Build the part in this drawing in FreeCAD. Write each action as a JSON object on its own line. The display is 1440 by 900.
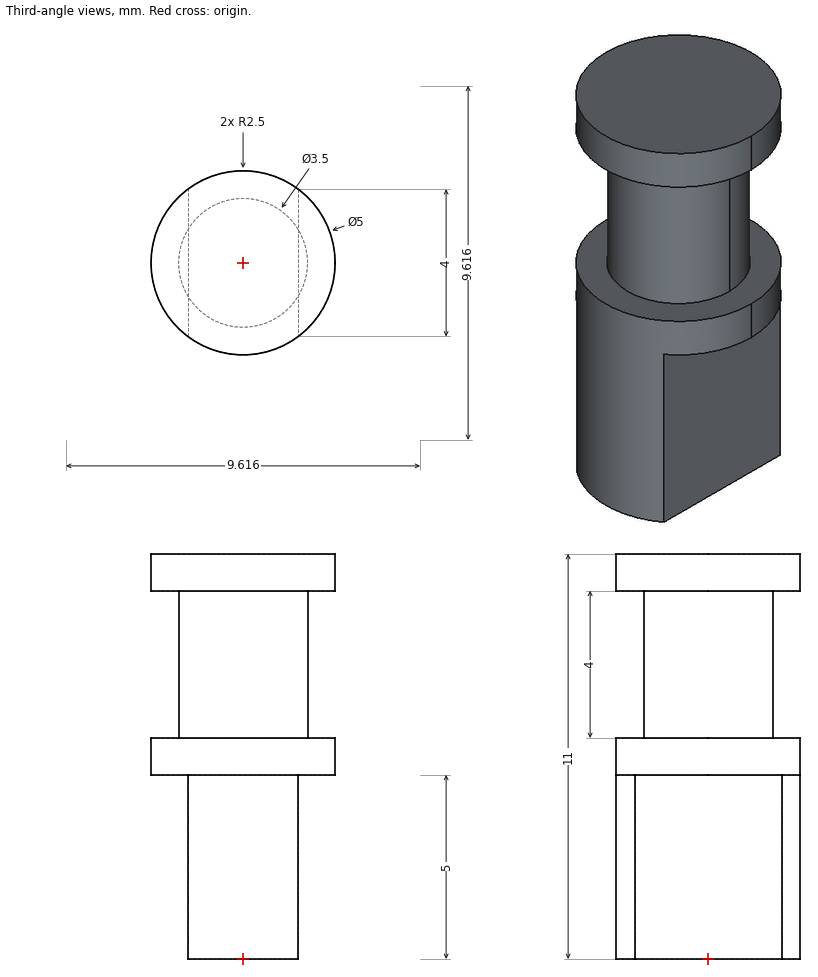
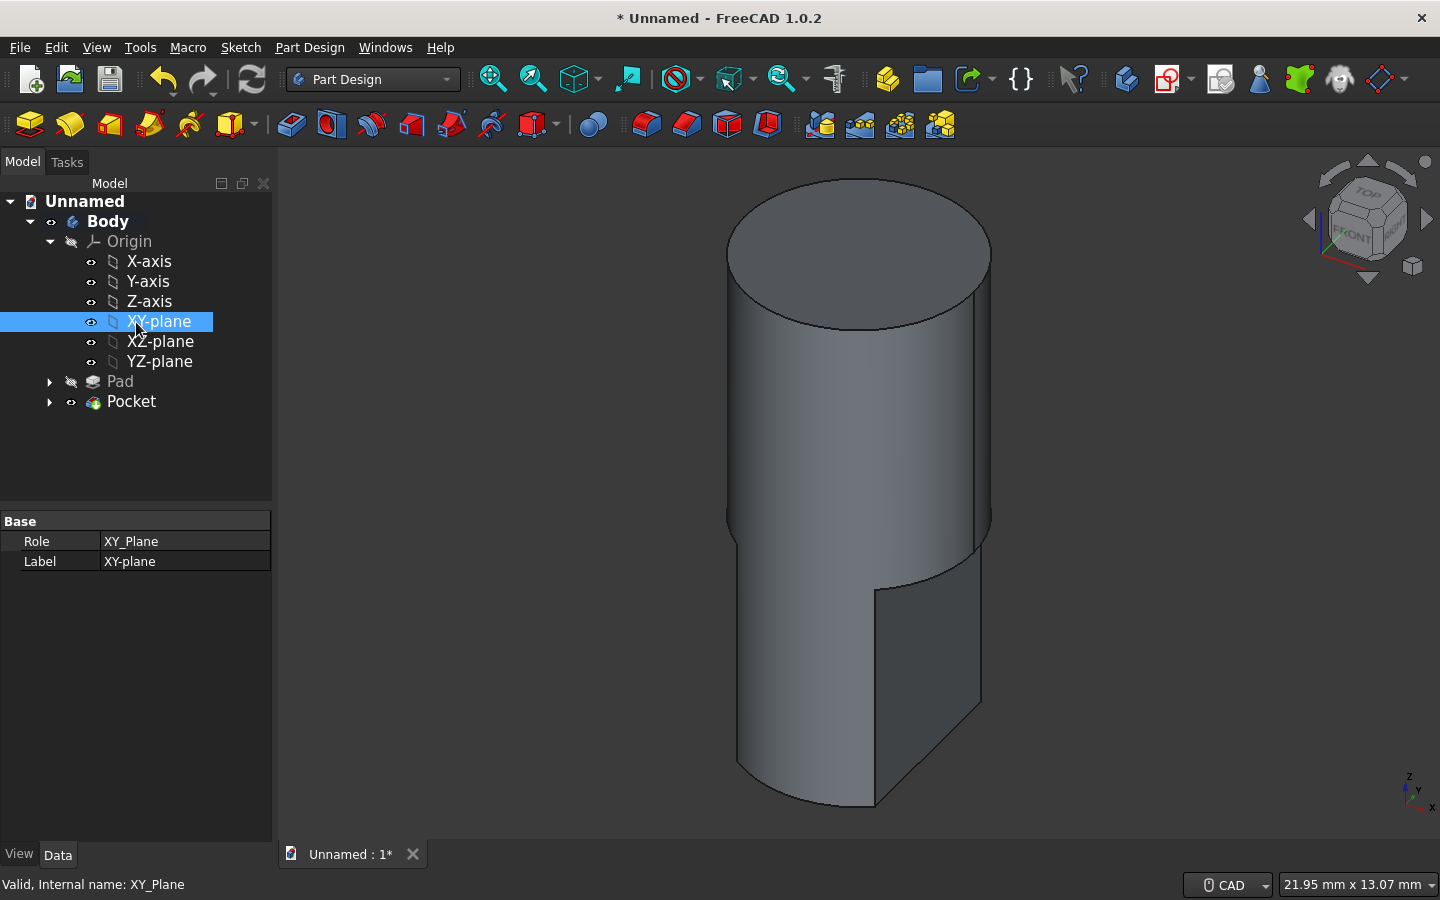
{"action": "left_click", "coordinate": [1380, 80]}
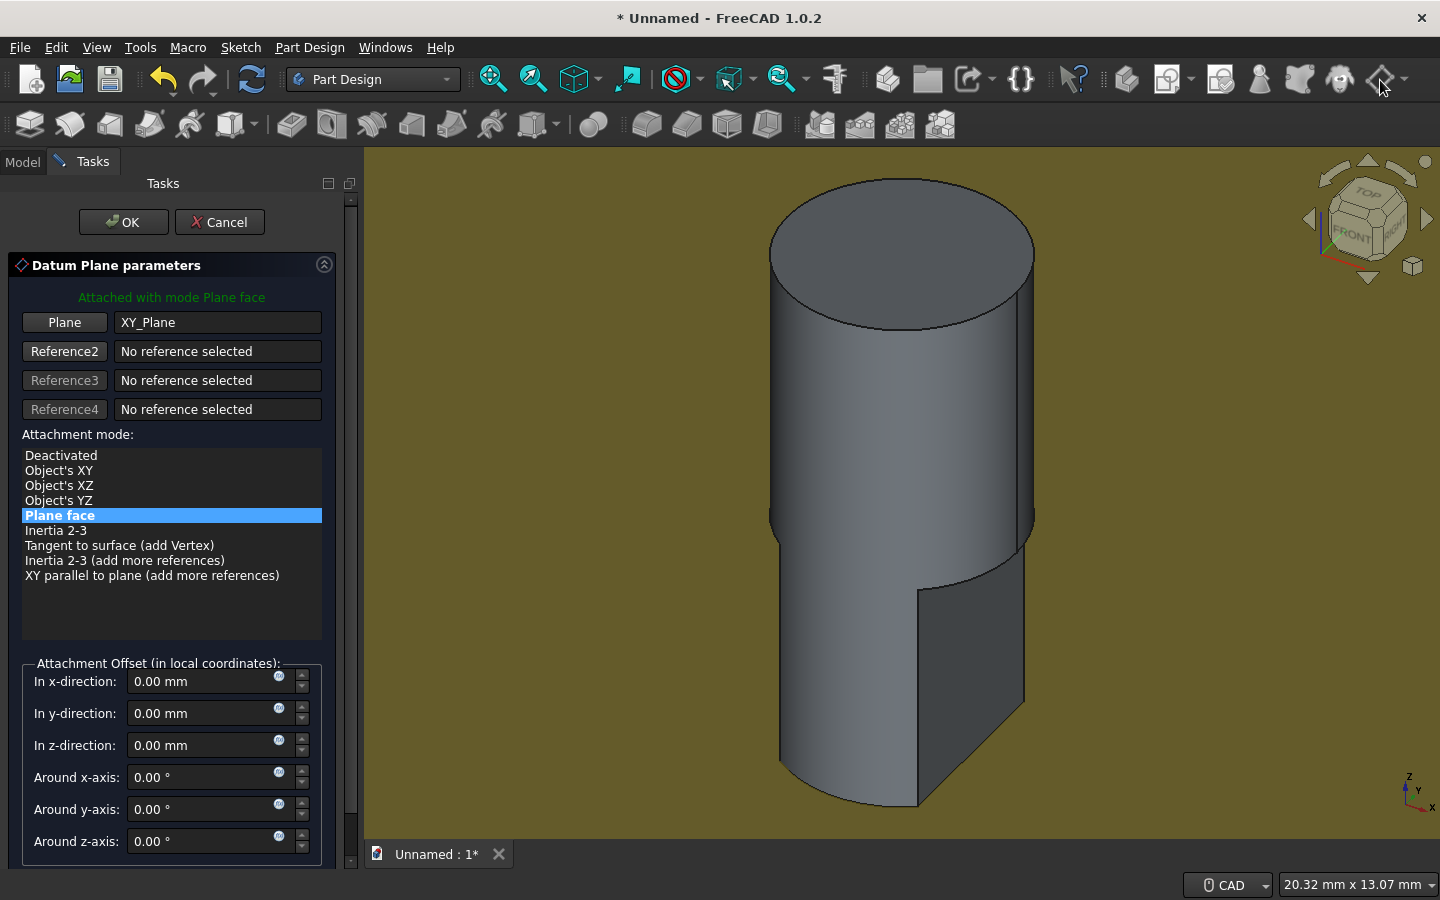
{"action": "triple_click", "coordinate": [210, 745]}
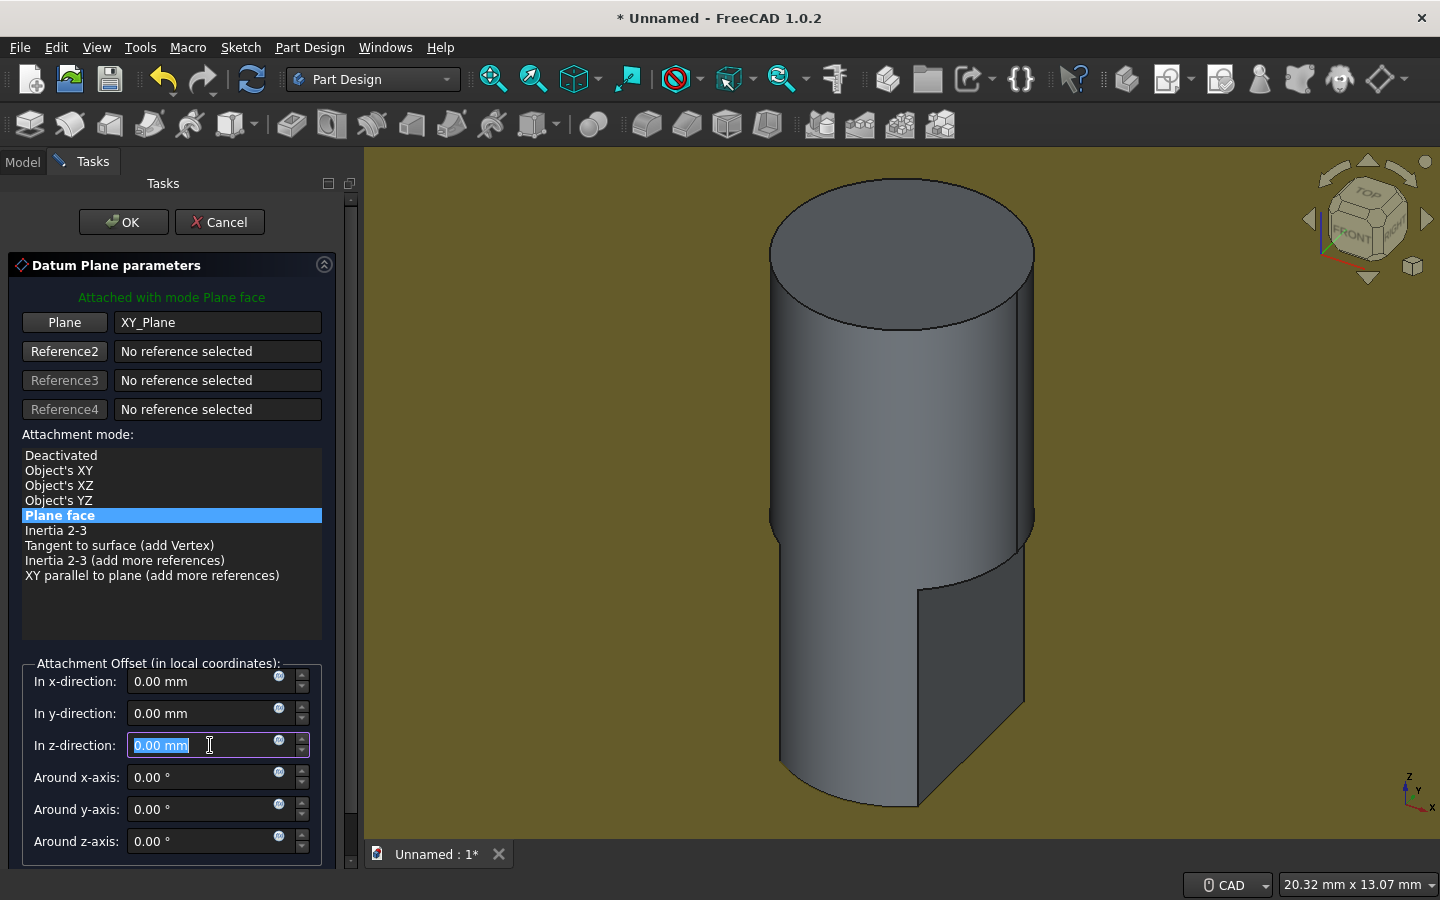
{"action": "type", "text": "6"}
{"action": "key", "text": "Tab"}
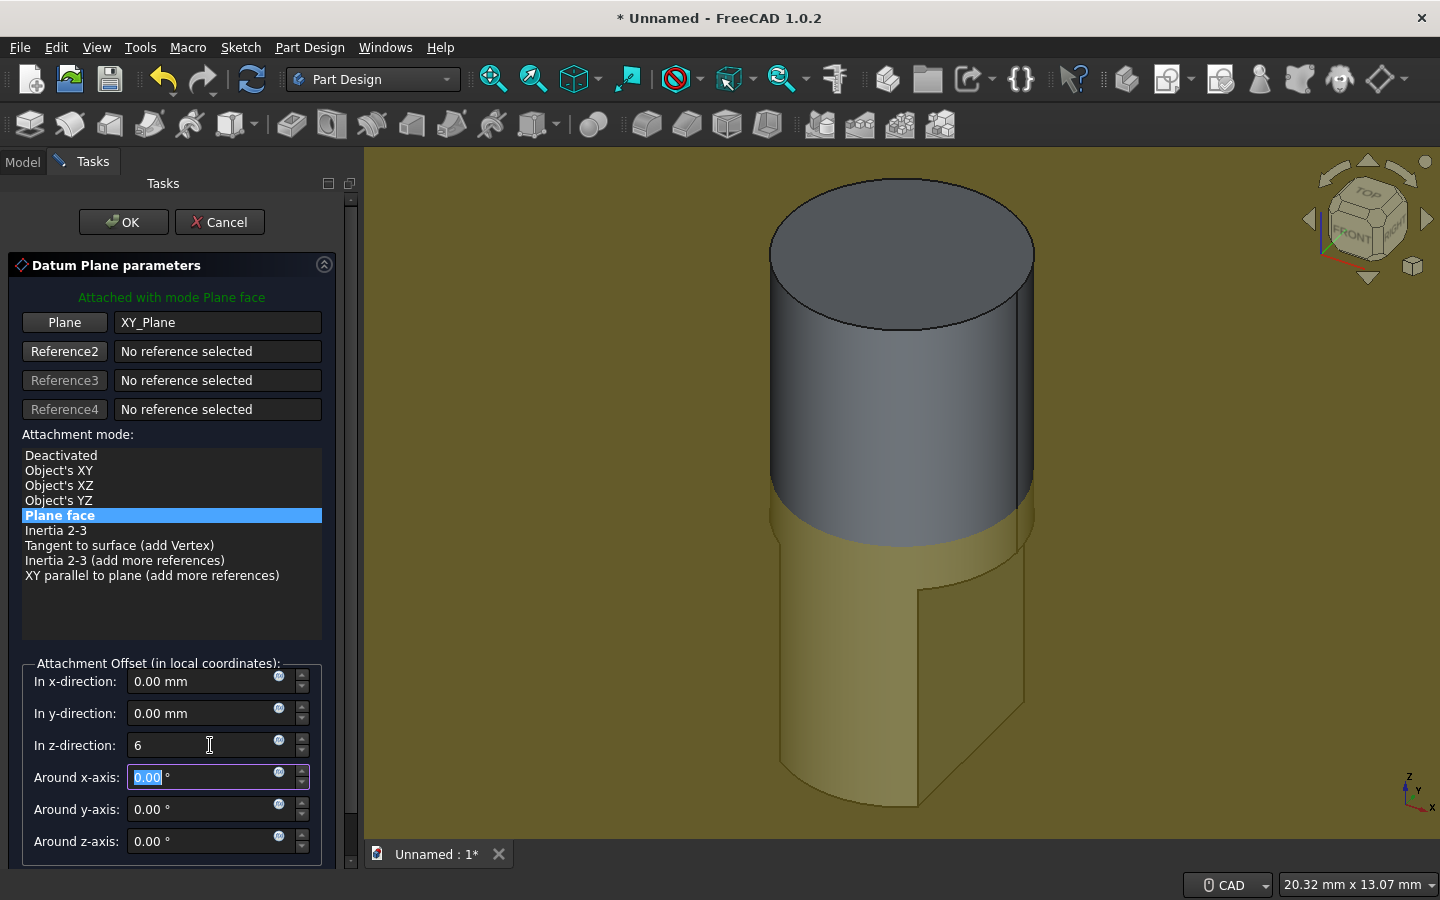
{"action": "left_click", "coordinate": [124, 222]}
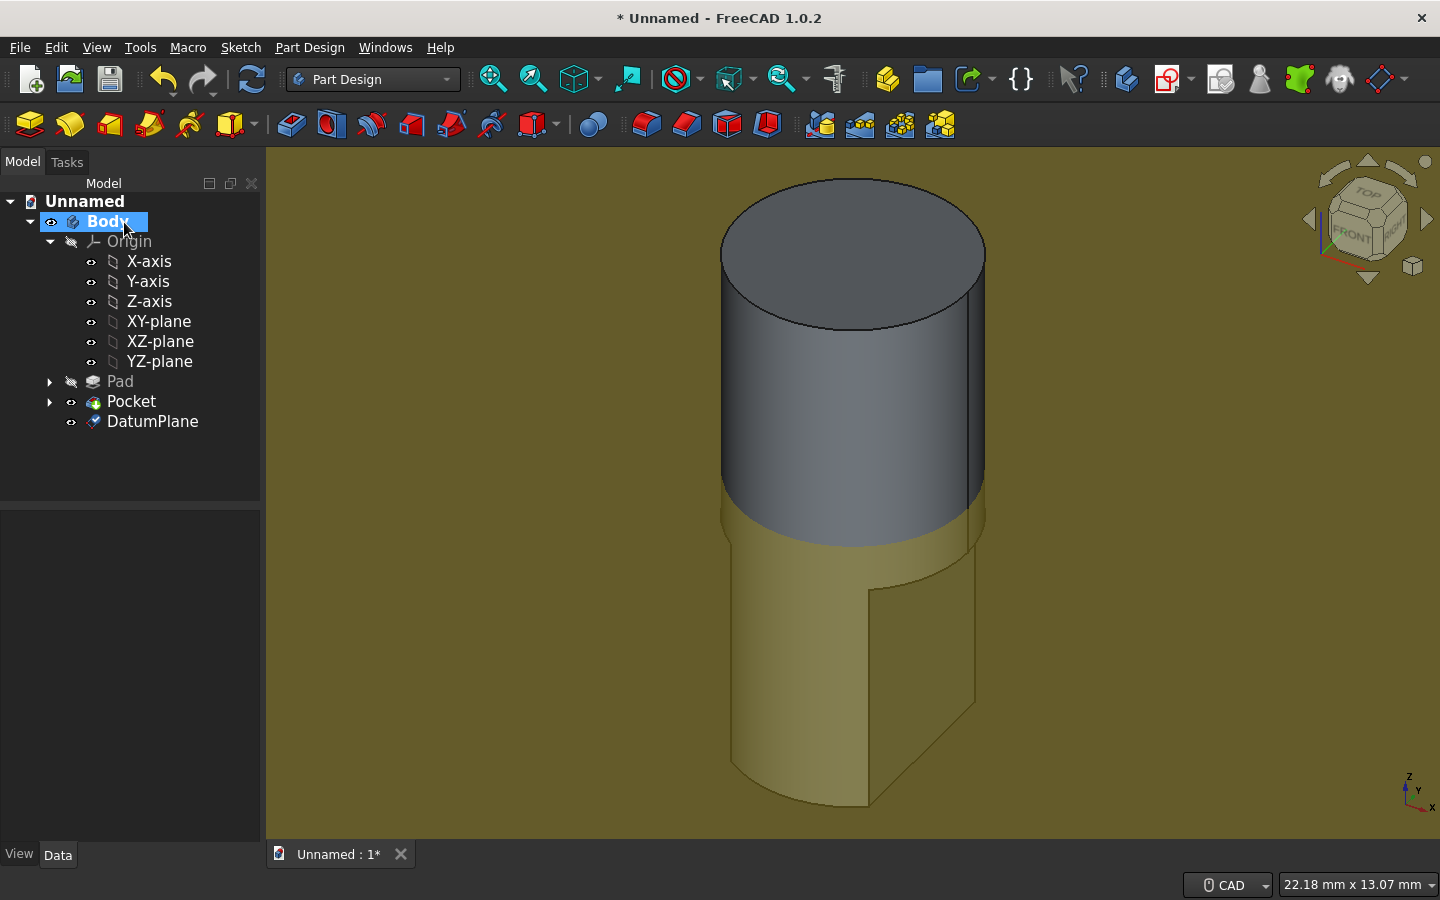
{"action": "left_click", "coordinate": [116, 422]}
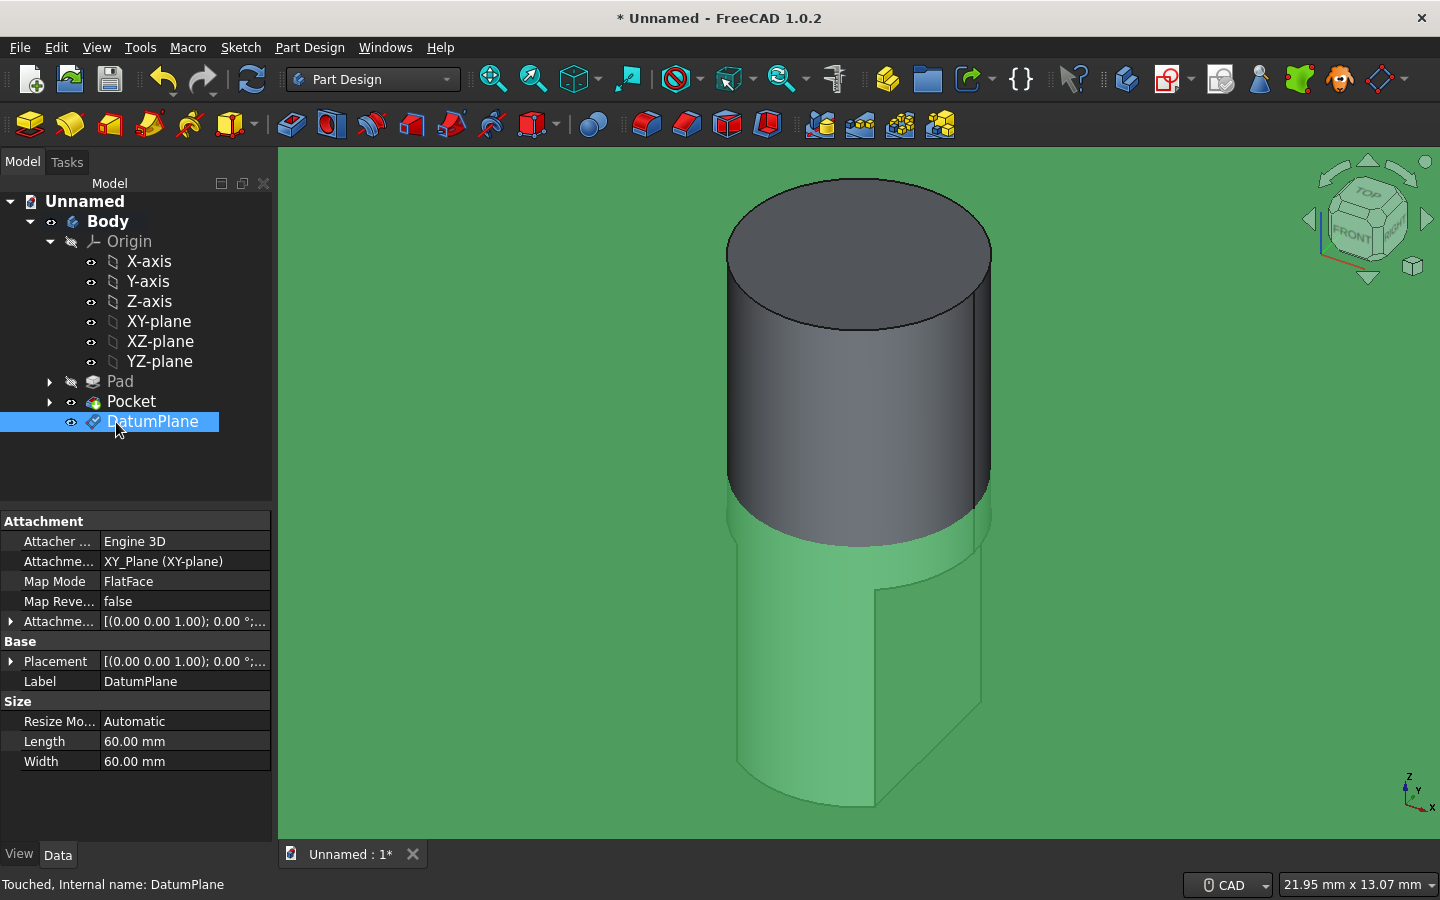
{"action": "left_click", "coordinate": [1168, 80]}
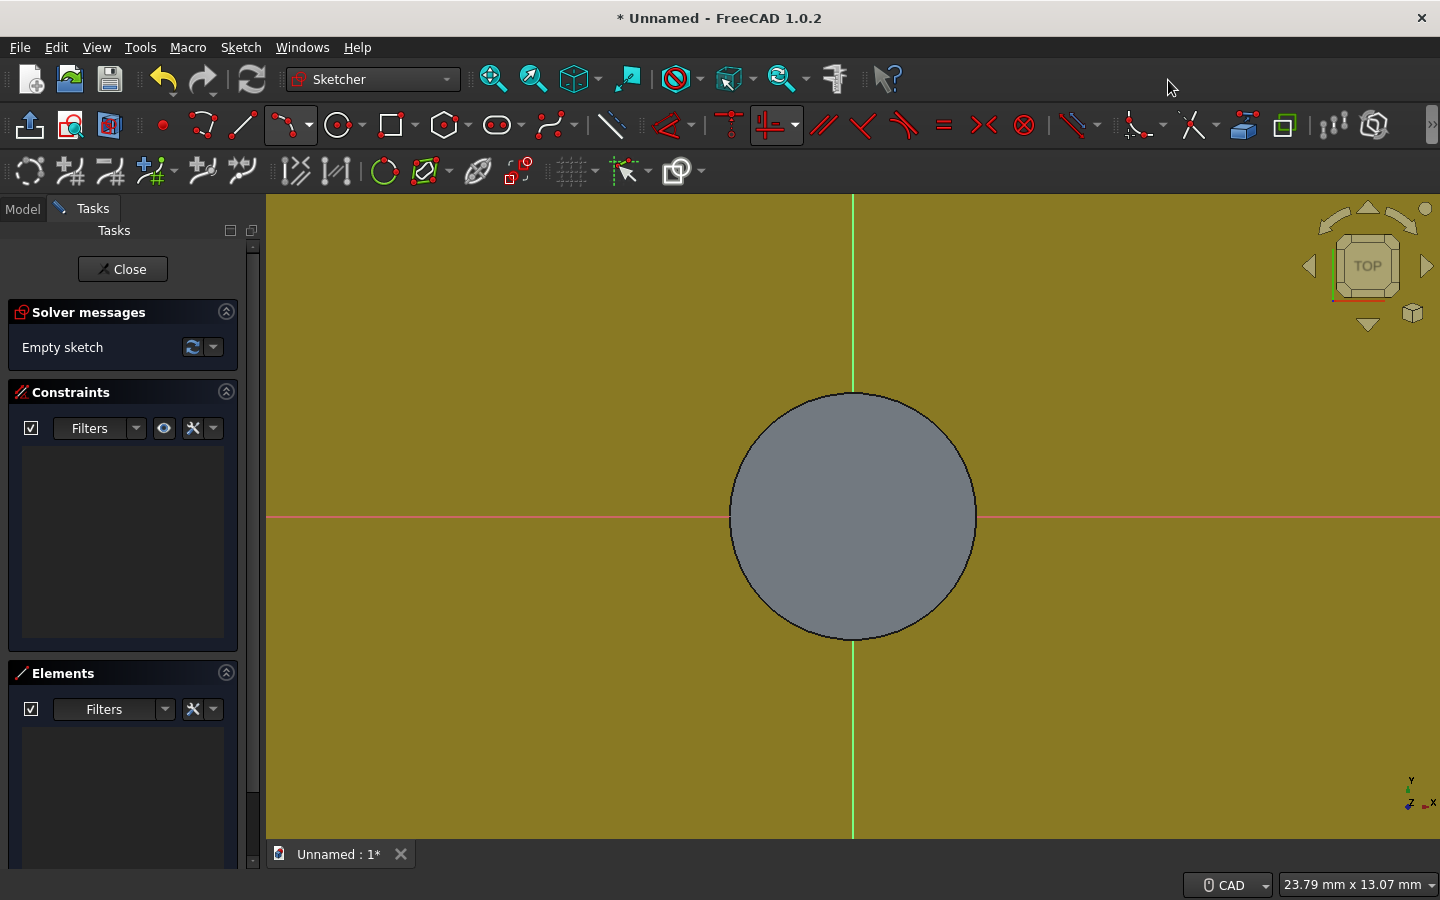
{"action": "left_click", "coordinate": [110, 126]}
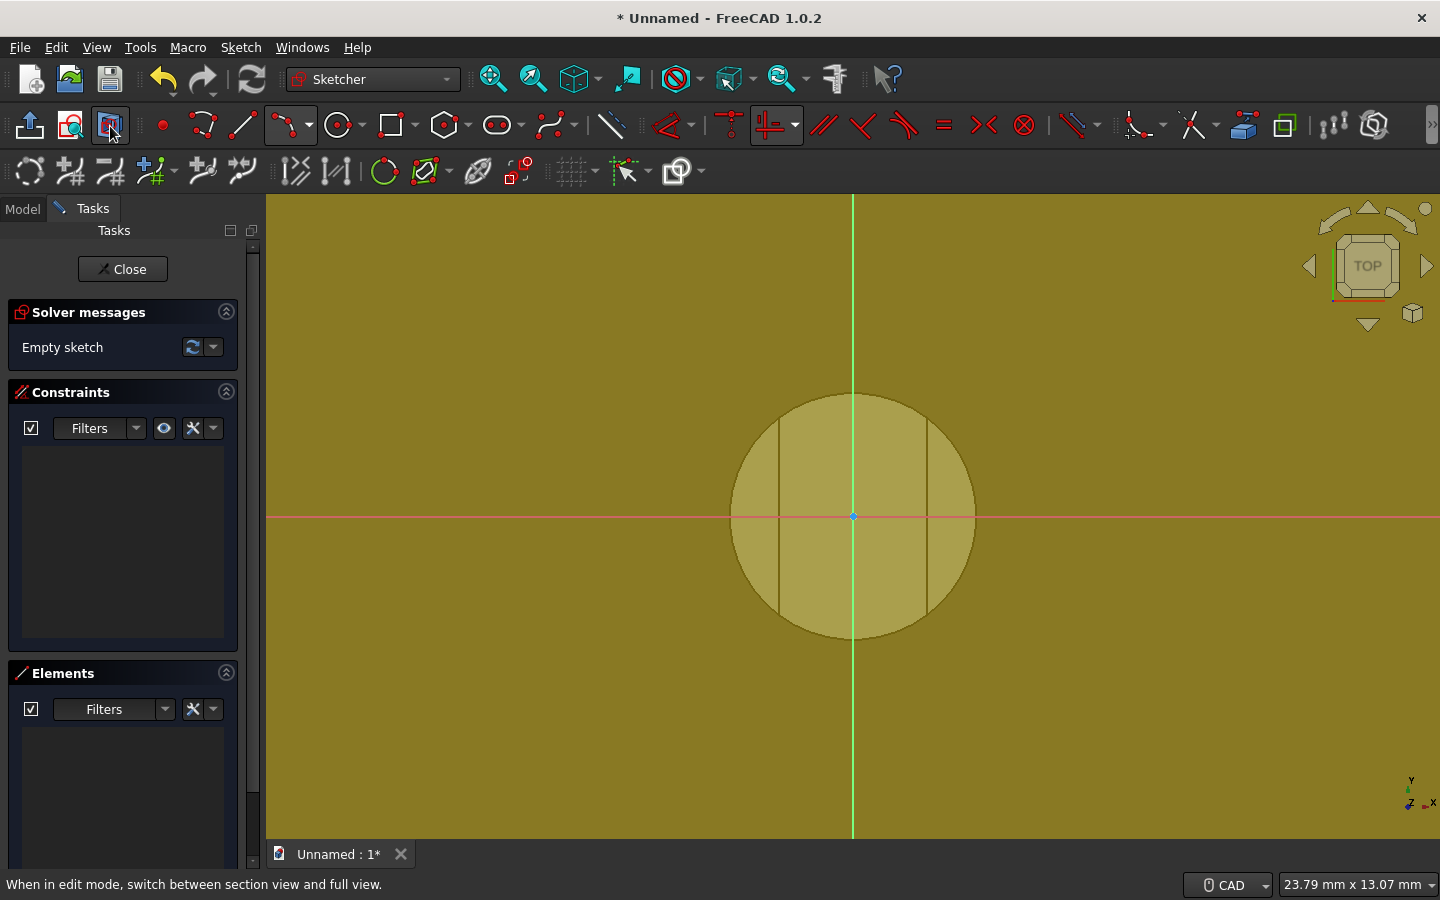
{"action": "scroll", "coordinate": [936, 516], "scroll_direction": "up", "scroll_amount": 3}